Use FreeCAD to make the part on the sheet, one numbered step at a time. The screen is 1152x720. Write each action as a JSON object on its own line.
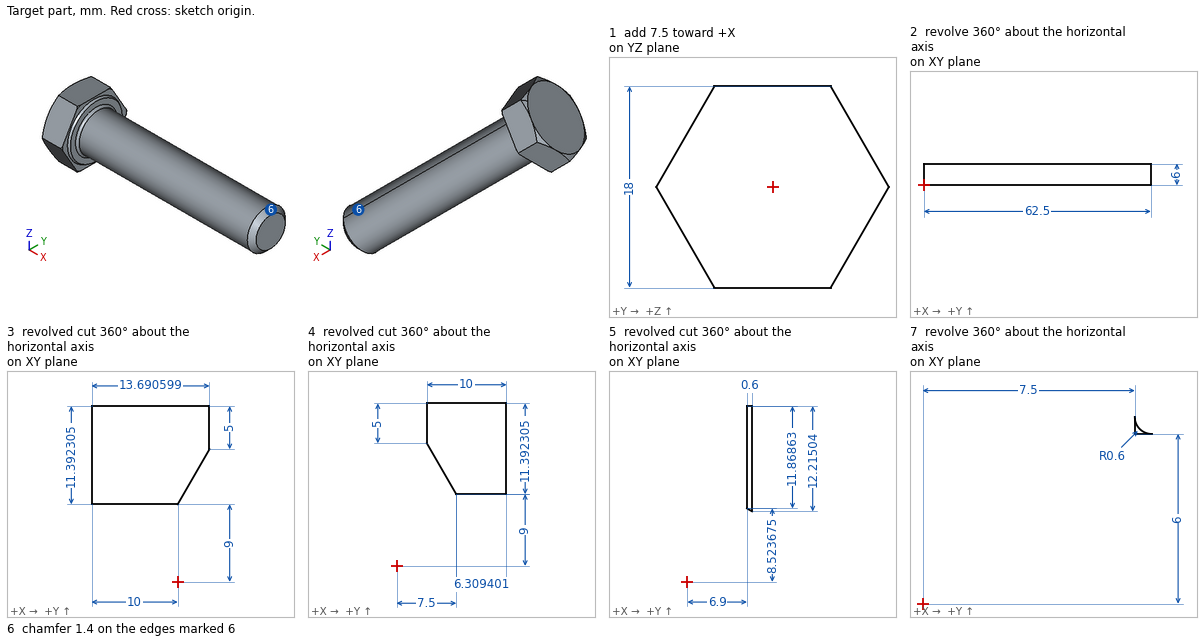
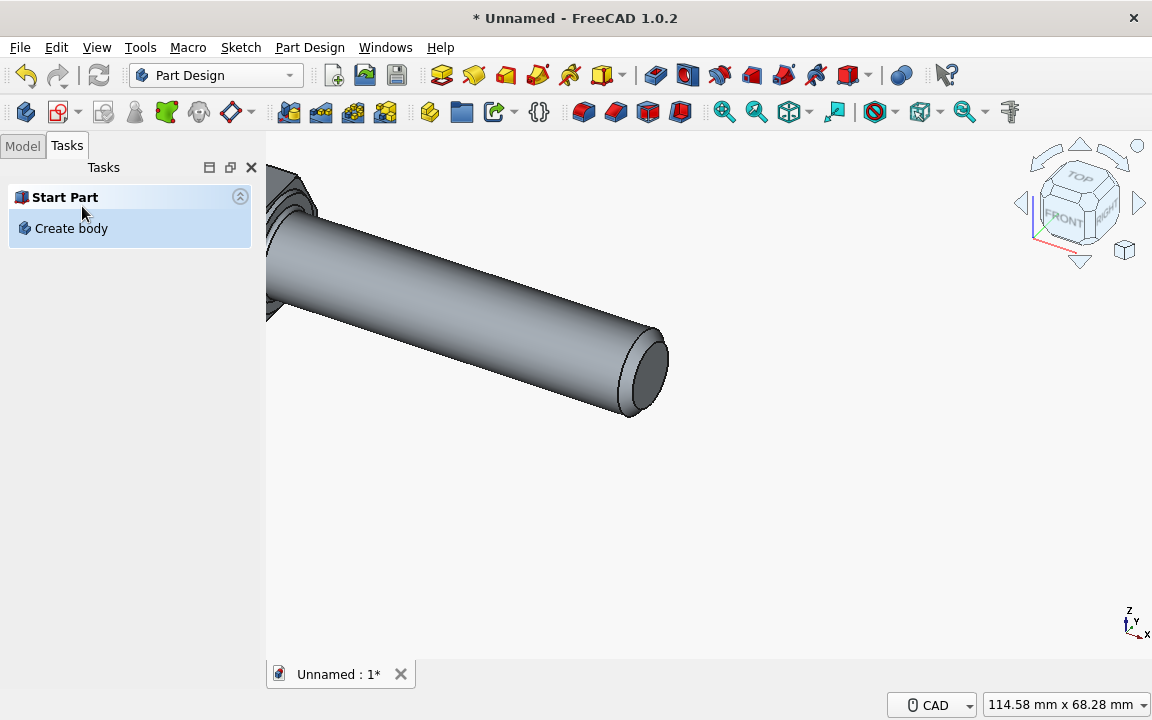
{"action": "key", "text": "0"}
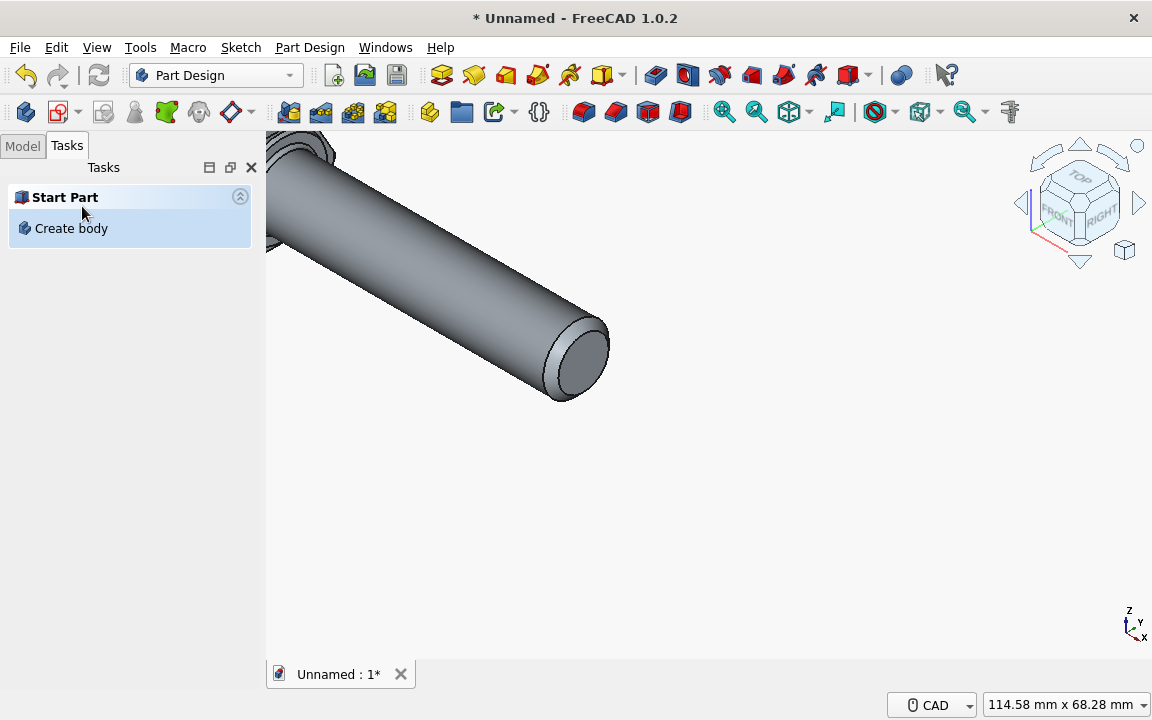
{"action": "key", "text": "v f"}